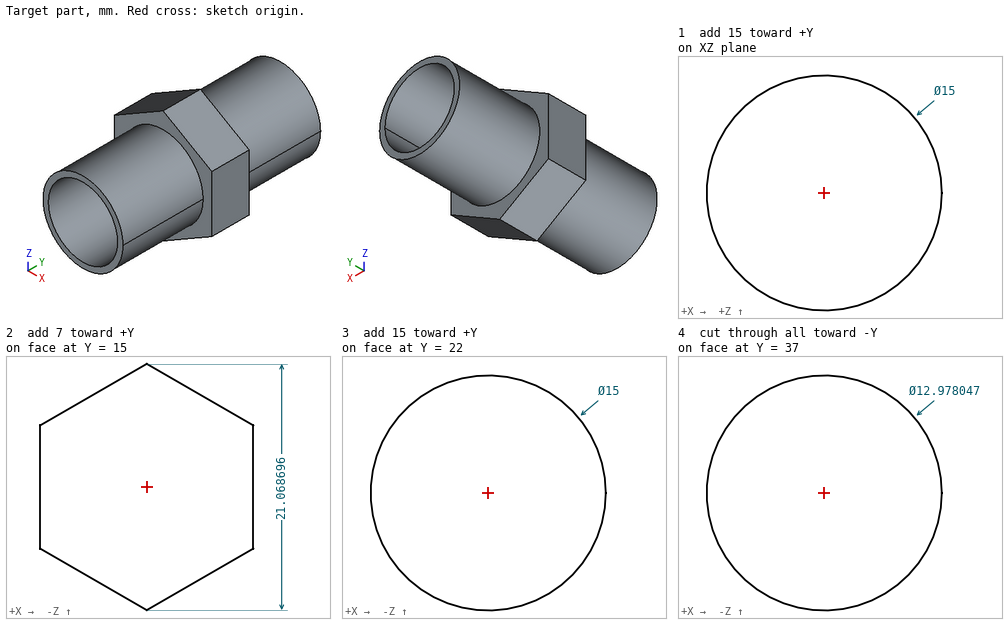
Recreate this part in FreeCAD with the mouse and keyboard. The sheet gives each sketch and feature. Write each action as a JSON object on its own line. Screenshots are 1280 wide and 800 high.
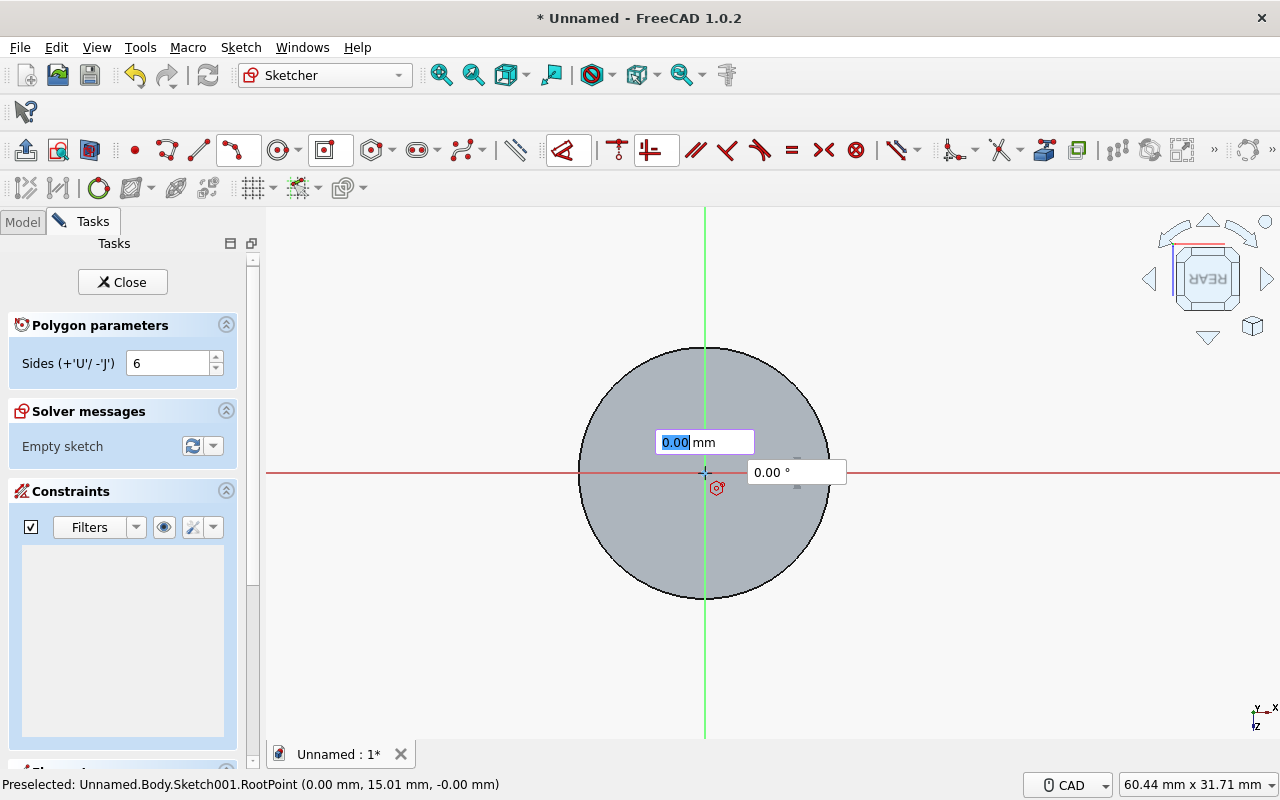
{"action": "left_click", "coordinate": [705, 650]}
{"action": "right_click", "coordinate": [705, 650]}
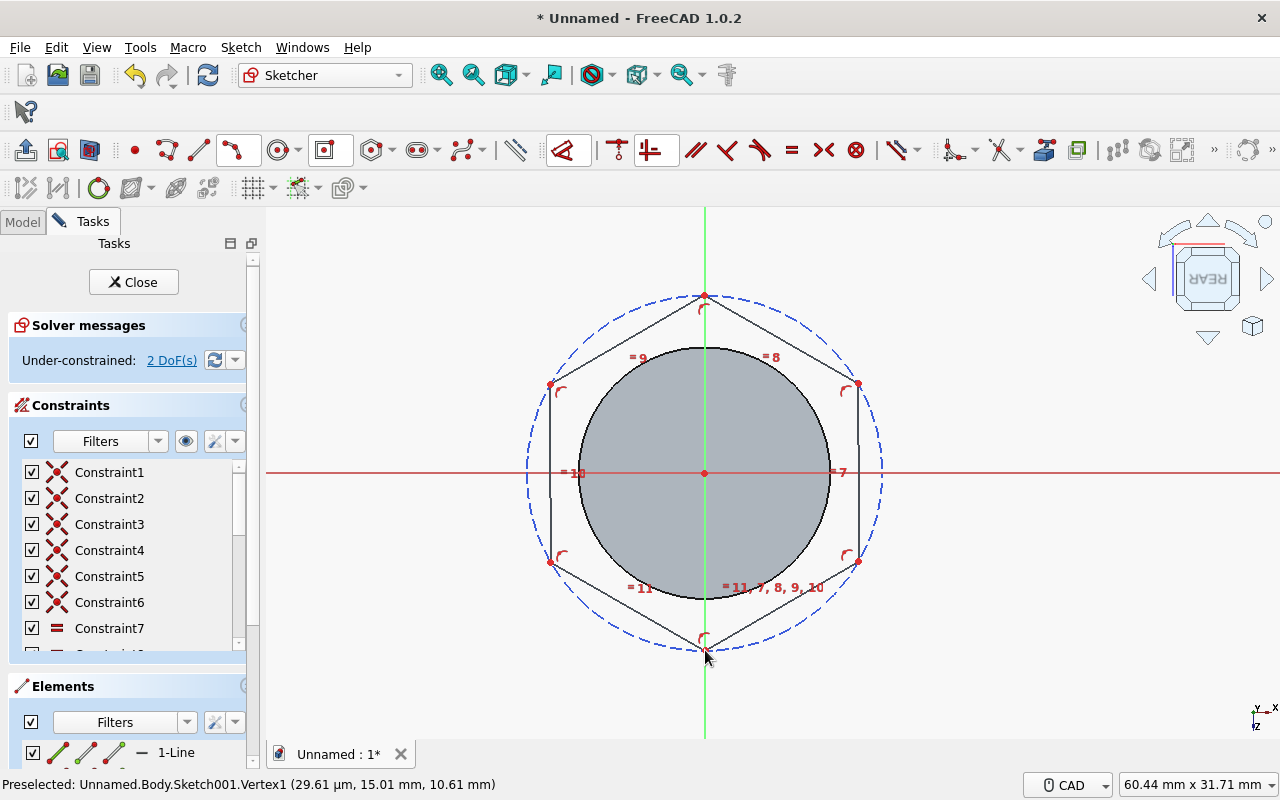
{"action": "left_click", "coordinate": [859, 508]}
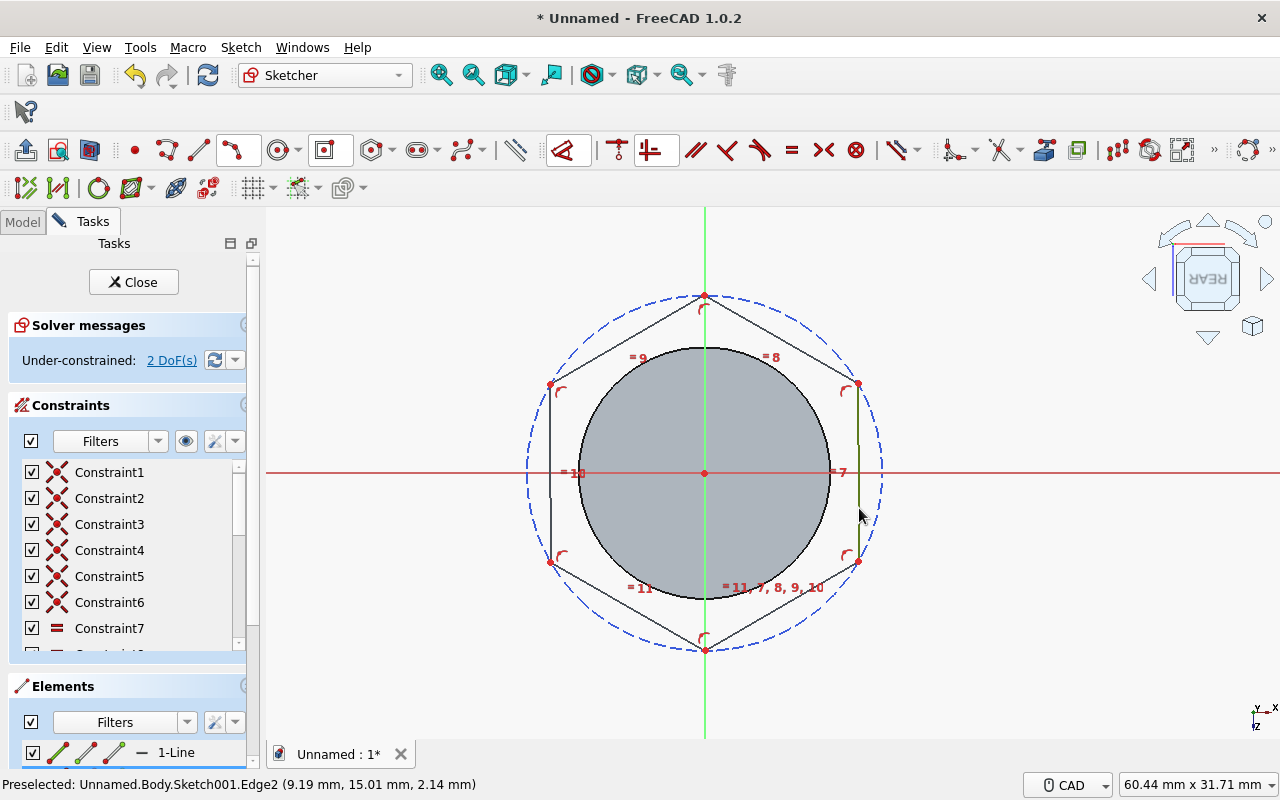
{"action": "left_click", "coordinate": [674, 150]}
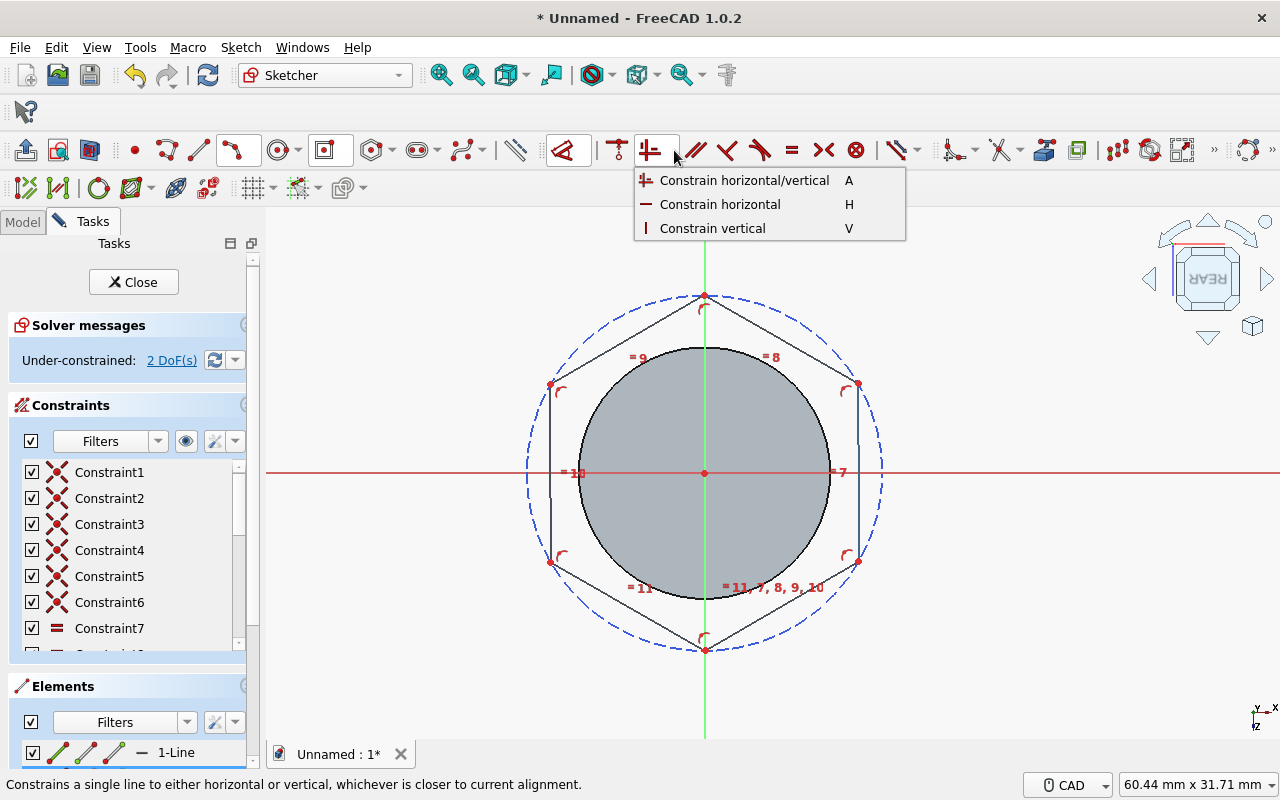
{"action": "left_click", "coordinate": [770, 228]}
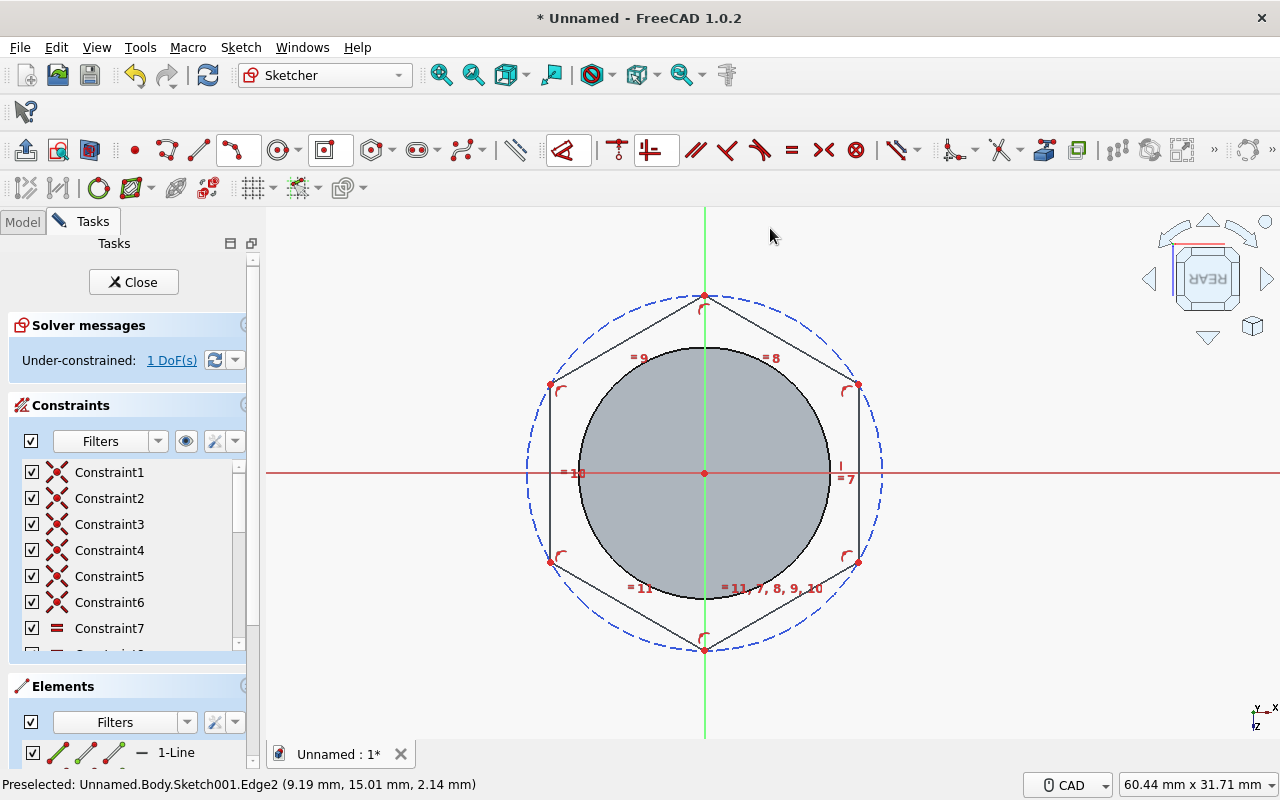
{"action": "left_click", "coordinate": [562, 150]}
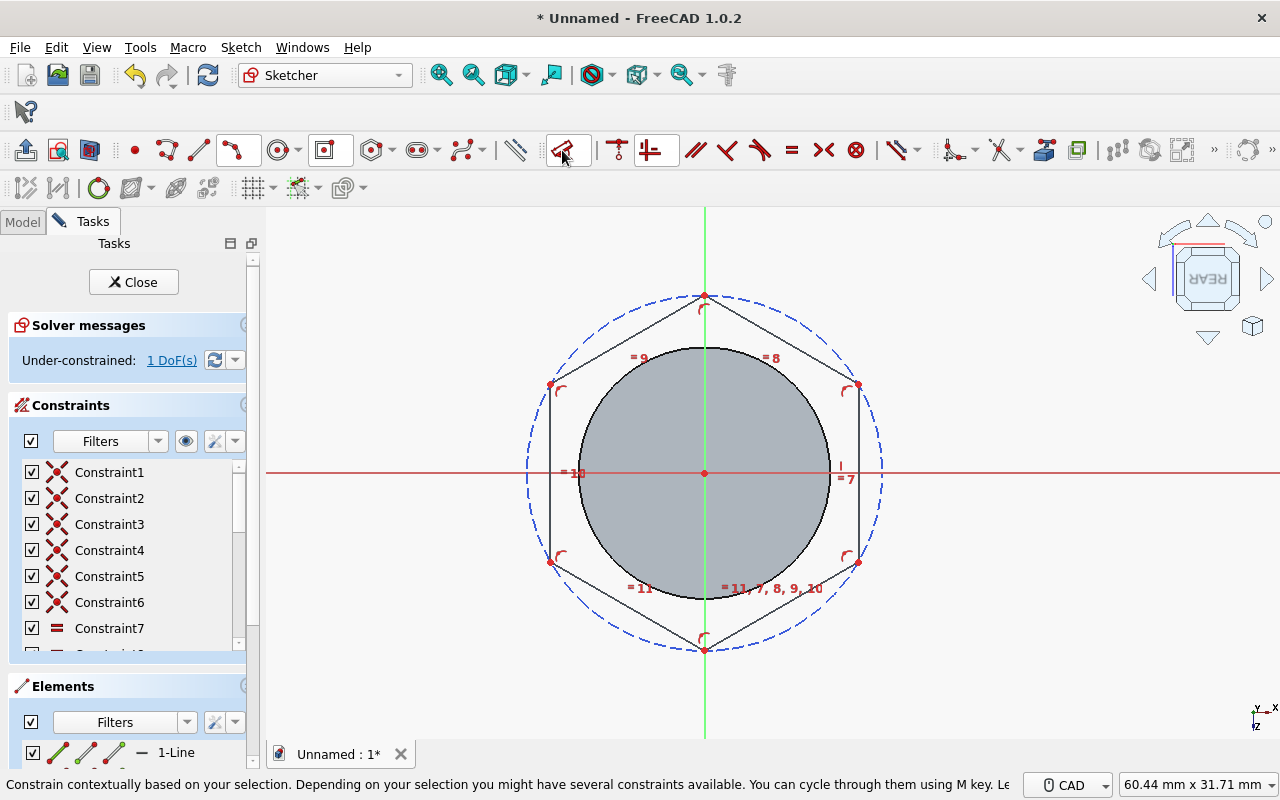
{"action": "left_click", "coordinate": [705, 651]}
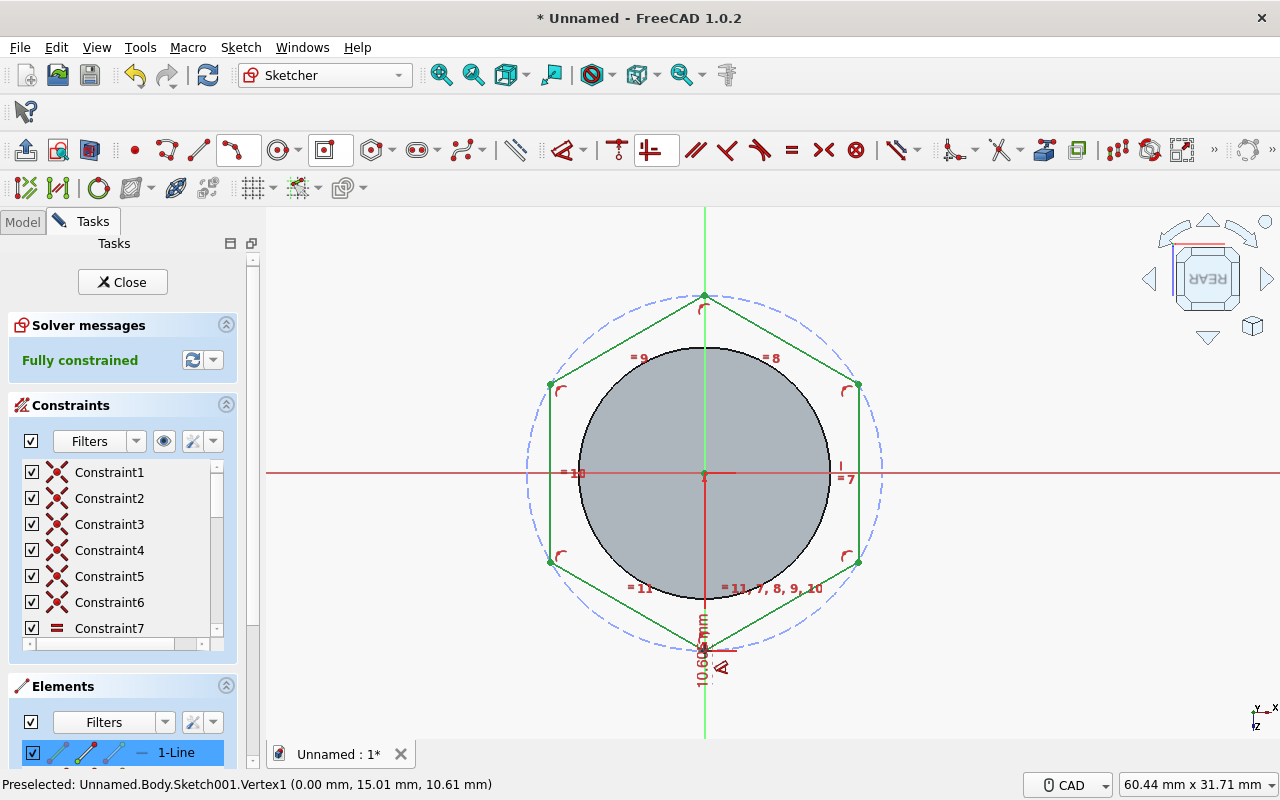
{"action": "left_click", "coordinate": [705, 295]}
{"action": "left_click", "coordinate": [739, 391]}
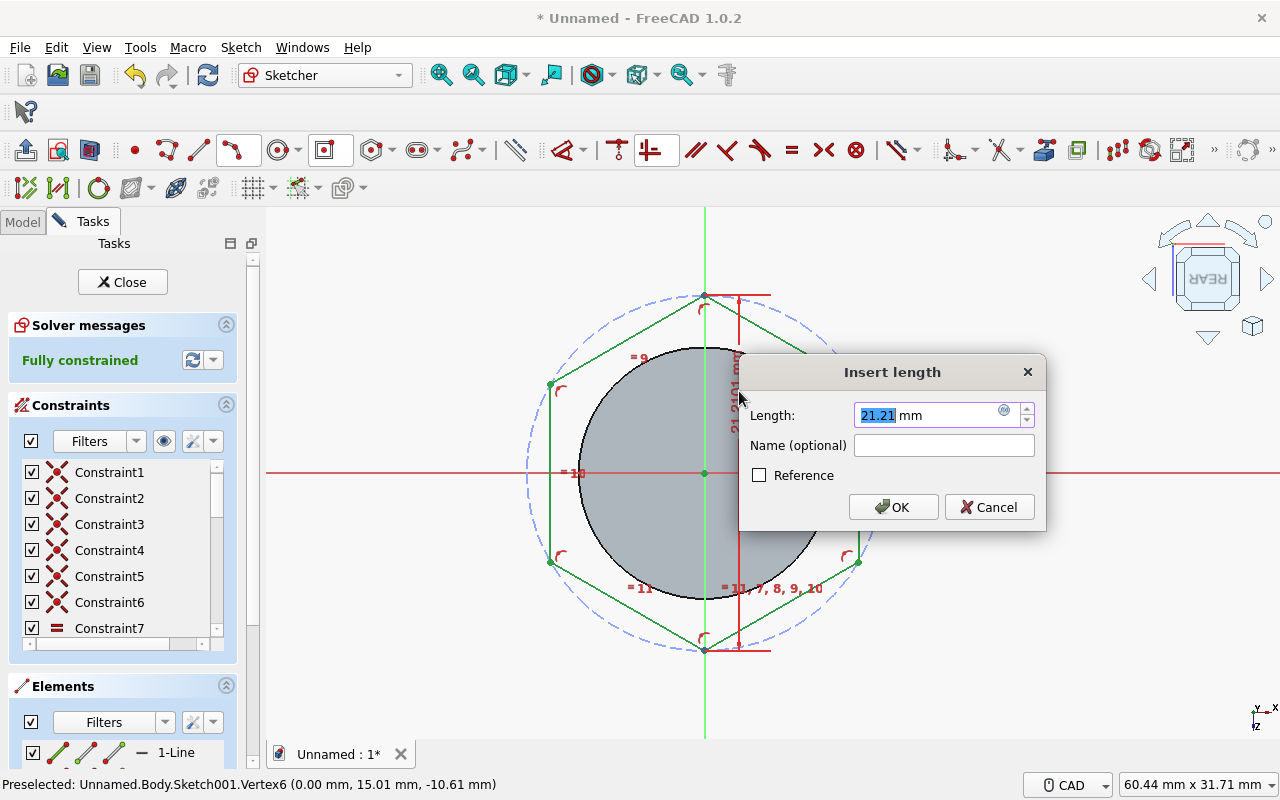
{"action": "type", "text": "21.068696"}
{"action": "key", "text": "Return"}
{"action": "key", "text": "Escape"}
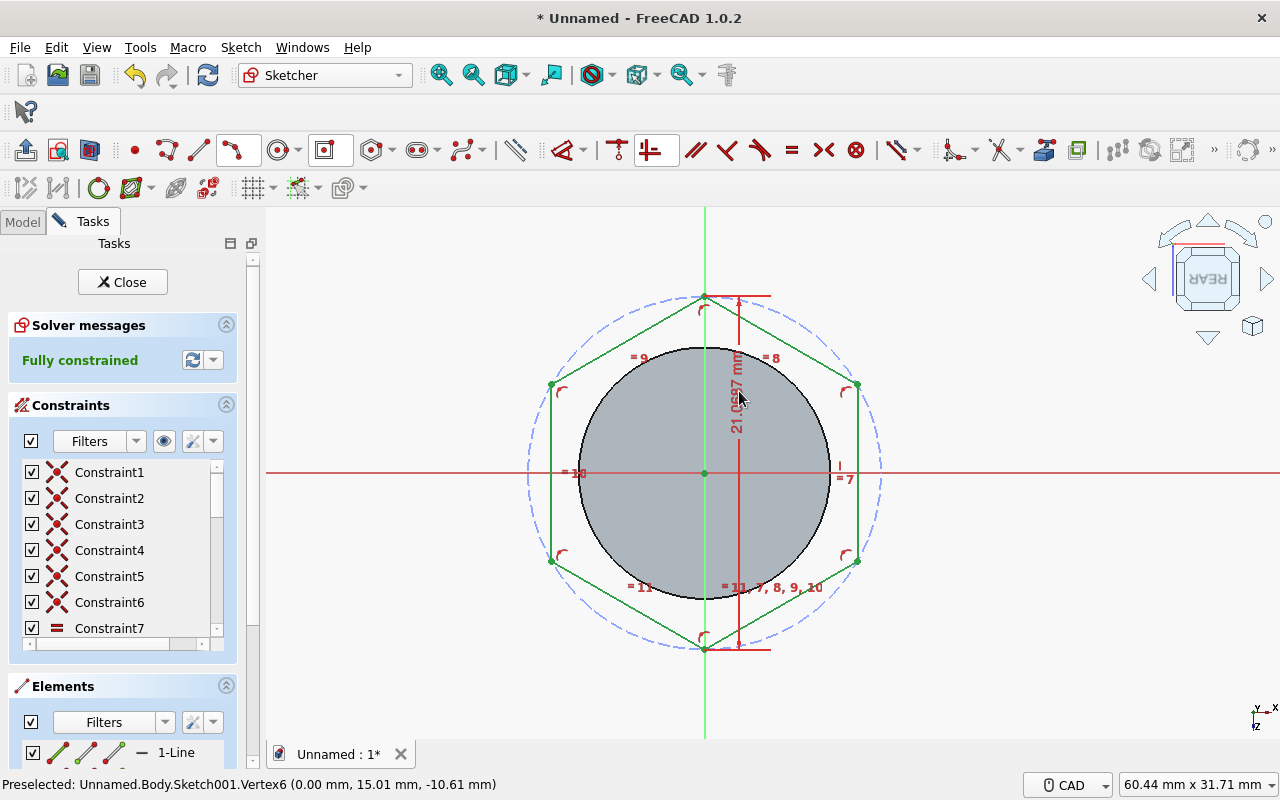
{"action": "left_click", "coordinate": [123, 282]}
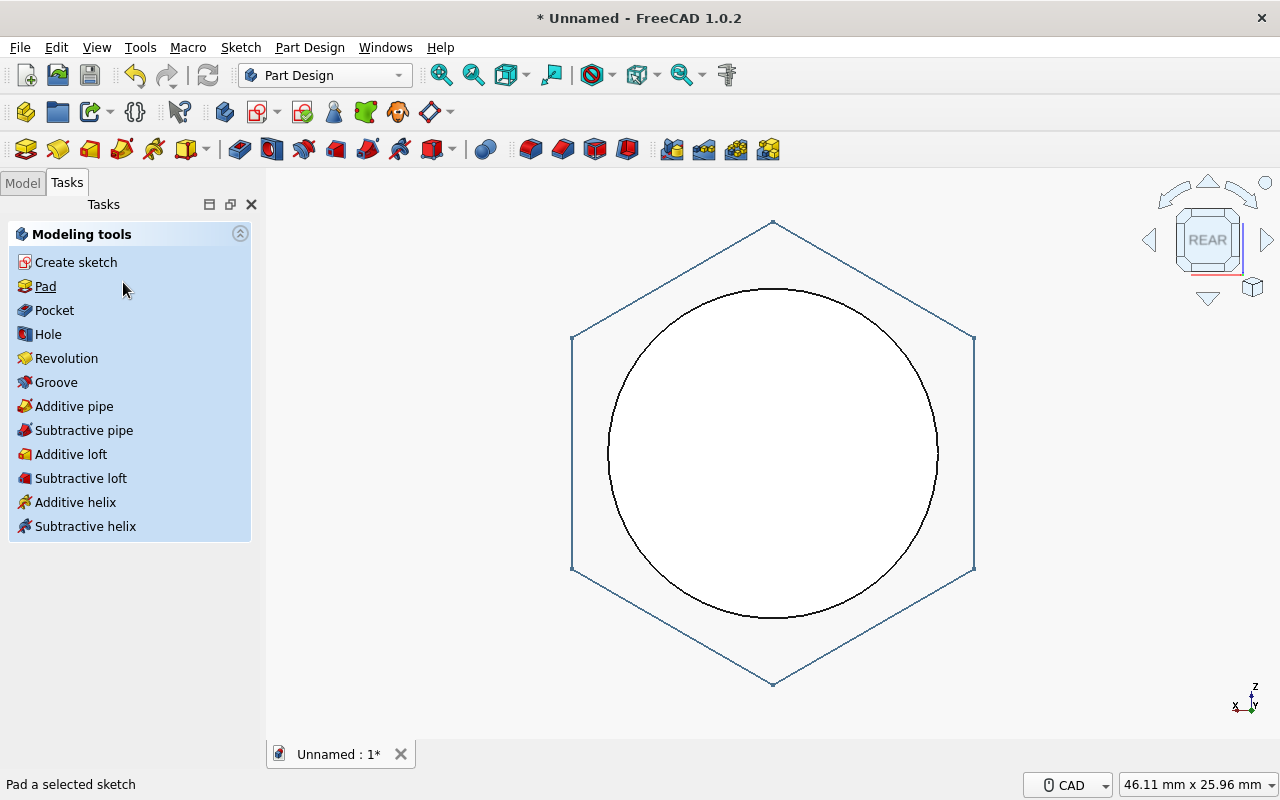
{"action": "left_click", "coordinate": [26, 150]}